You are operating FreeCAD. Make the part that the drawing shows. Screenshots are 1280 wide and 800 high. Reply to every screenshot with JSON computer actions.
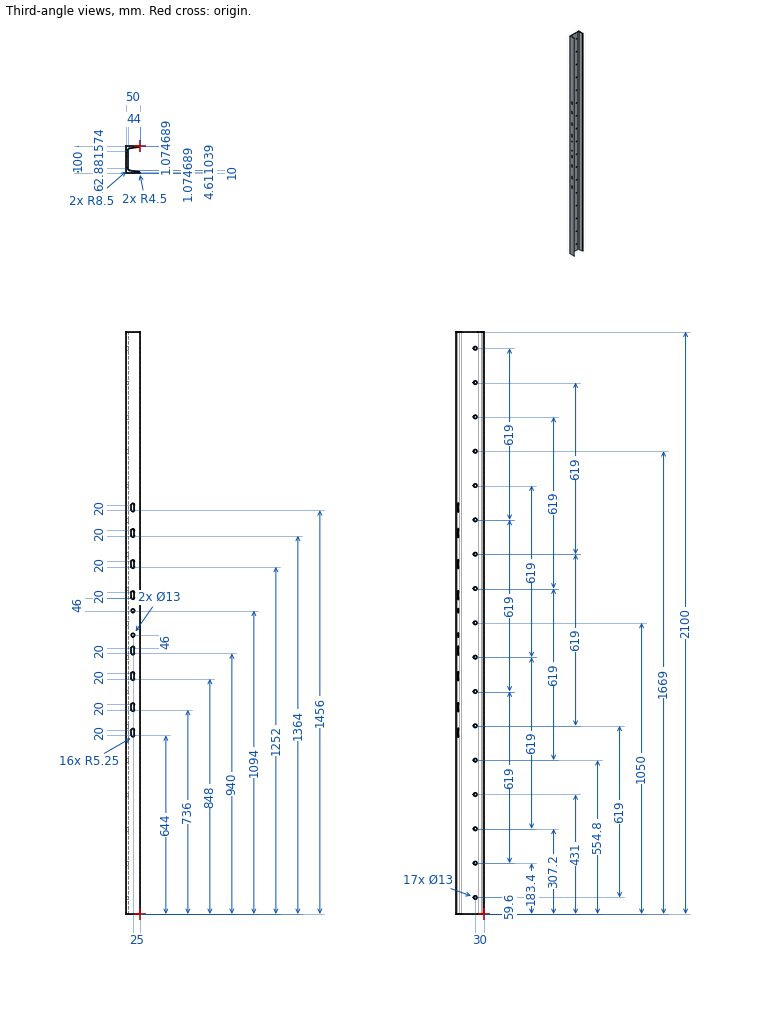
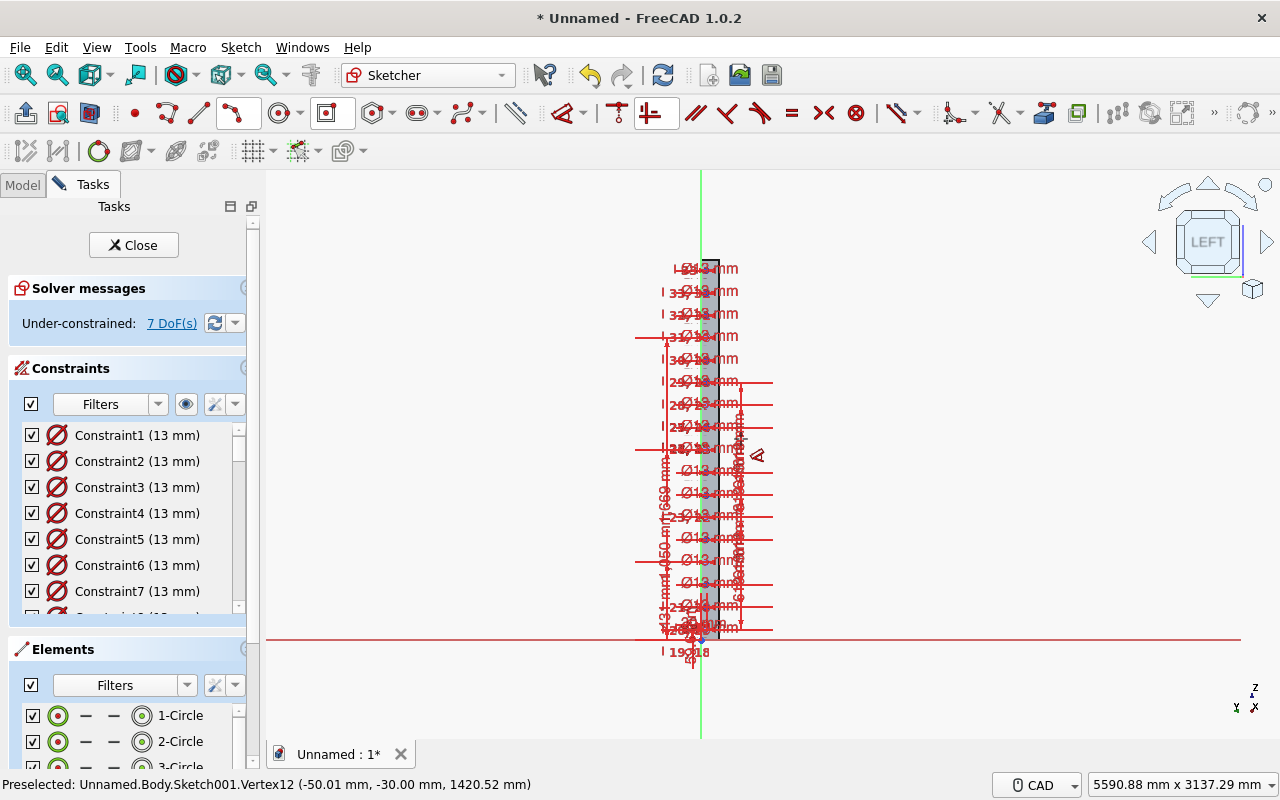
{"action": "left_click", "coordinate": [707, 473]}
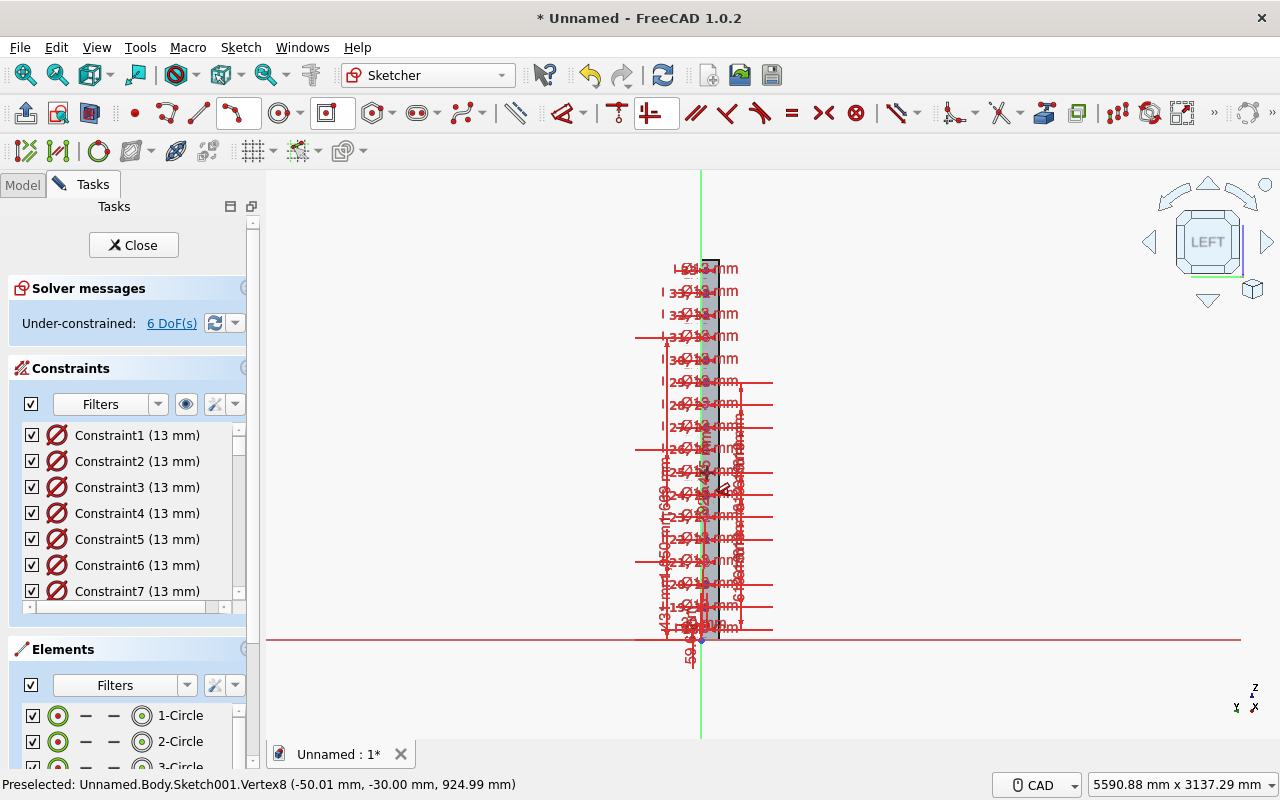
{"action": "left_click", "coordinate": [707, 361]}
{"action": "left_click", "coordinate": [741, 417]}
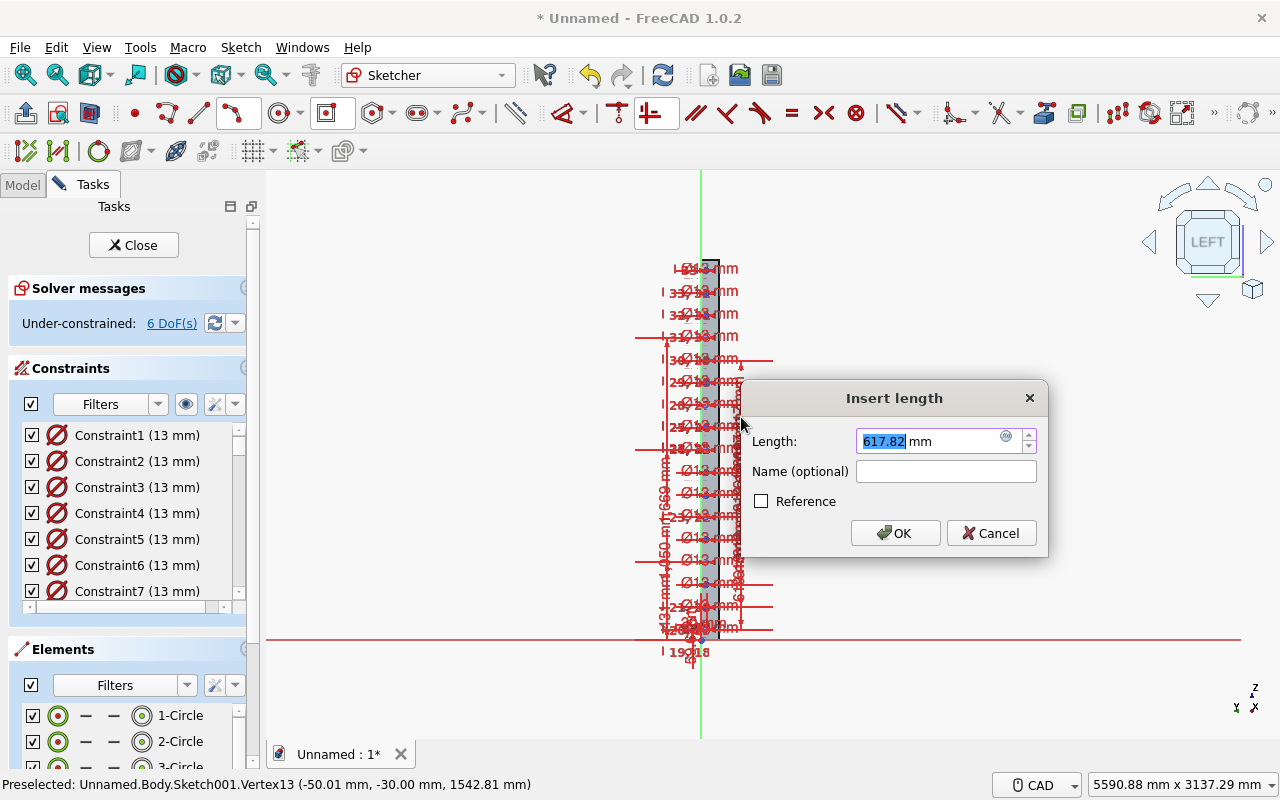
{"action": "type", "text": "619"}
{"action": "key", "text": "Return"}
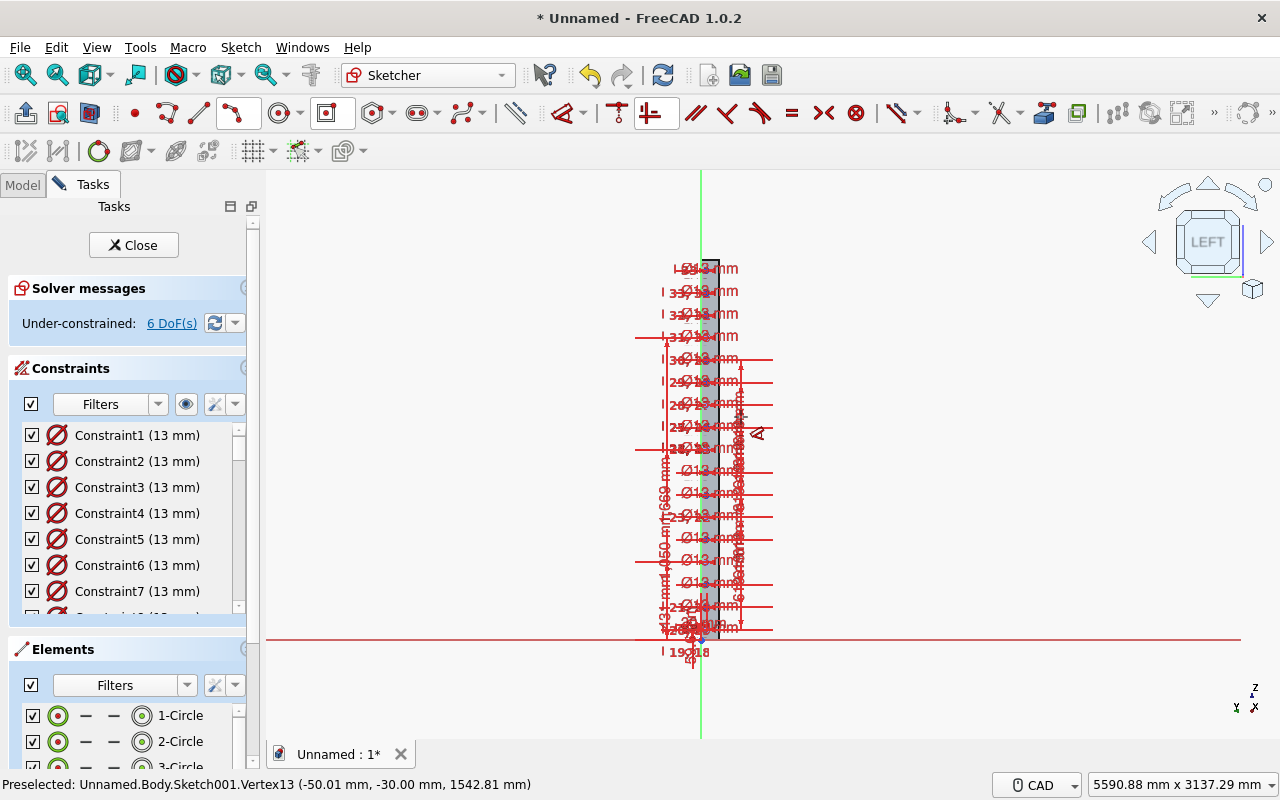
{"action": "left_click", "coordinate": [707, 428]}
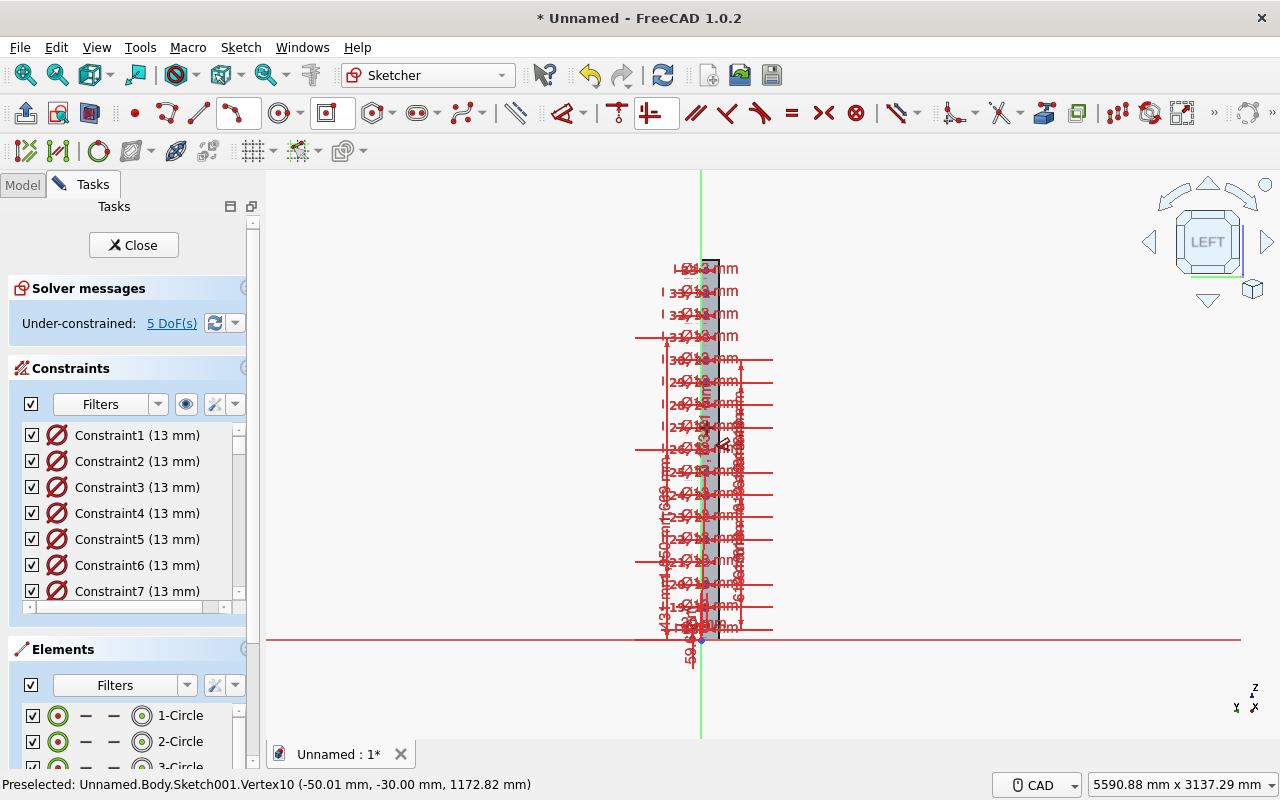
{"action": "left_click", "coordinate": [707, 316]}
{"action": "left_click", "coordinate": [741, 372]}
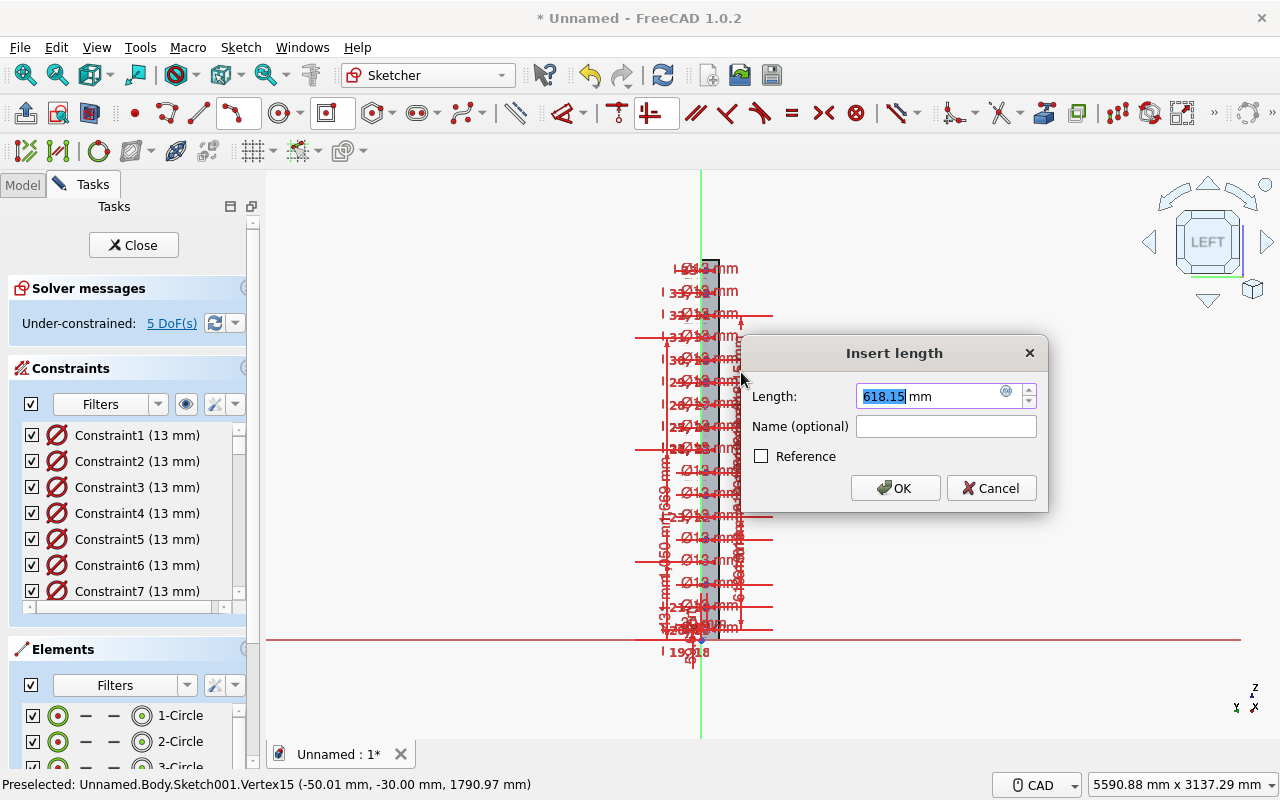
{"action": "type", "text": "619"}
{"action": "key", "text": "Return"}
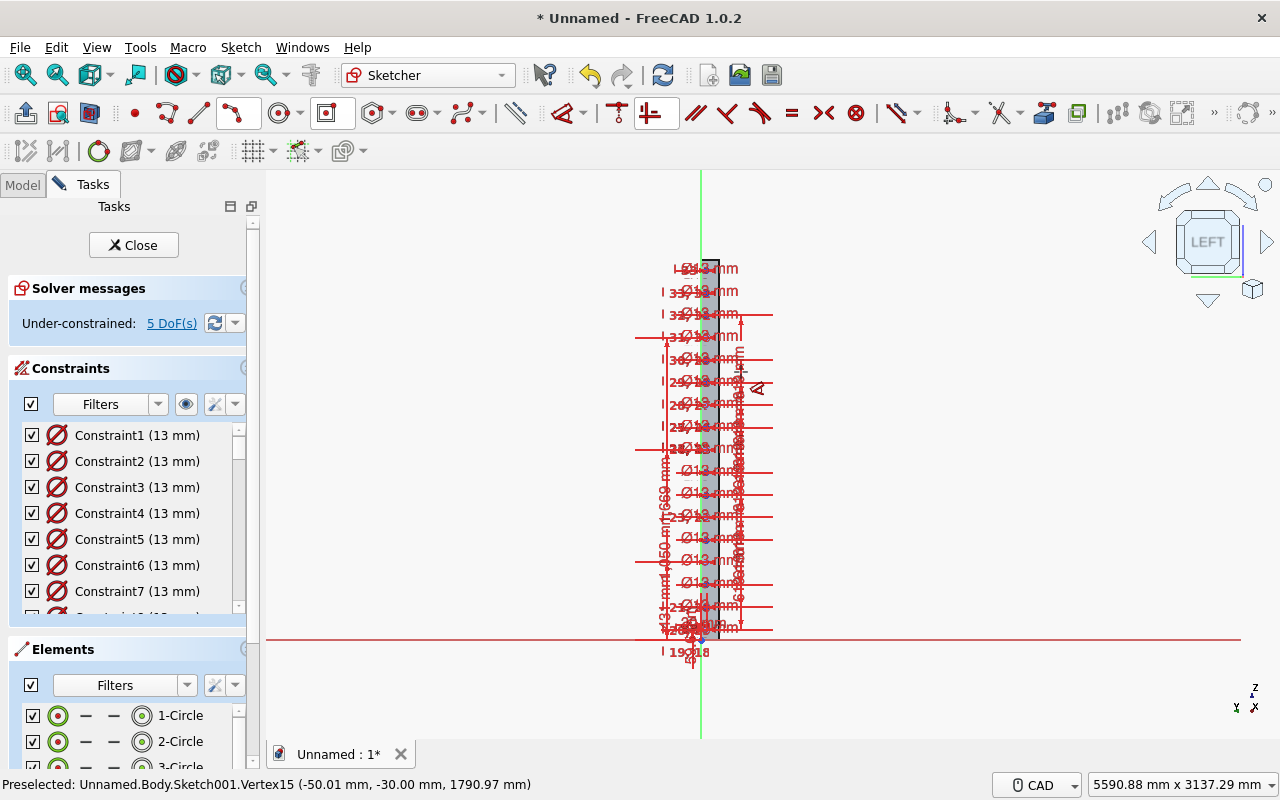
{"action": "left_click", "coordinate": [707, 405]}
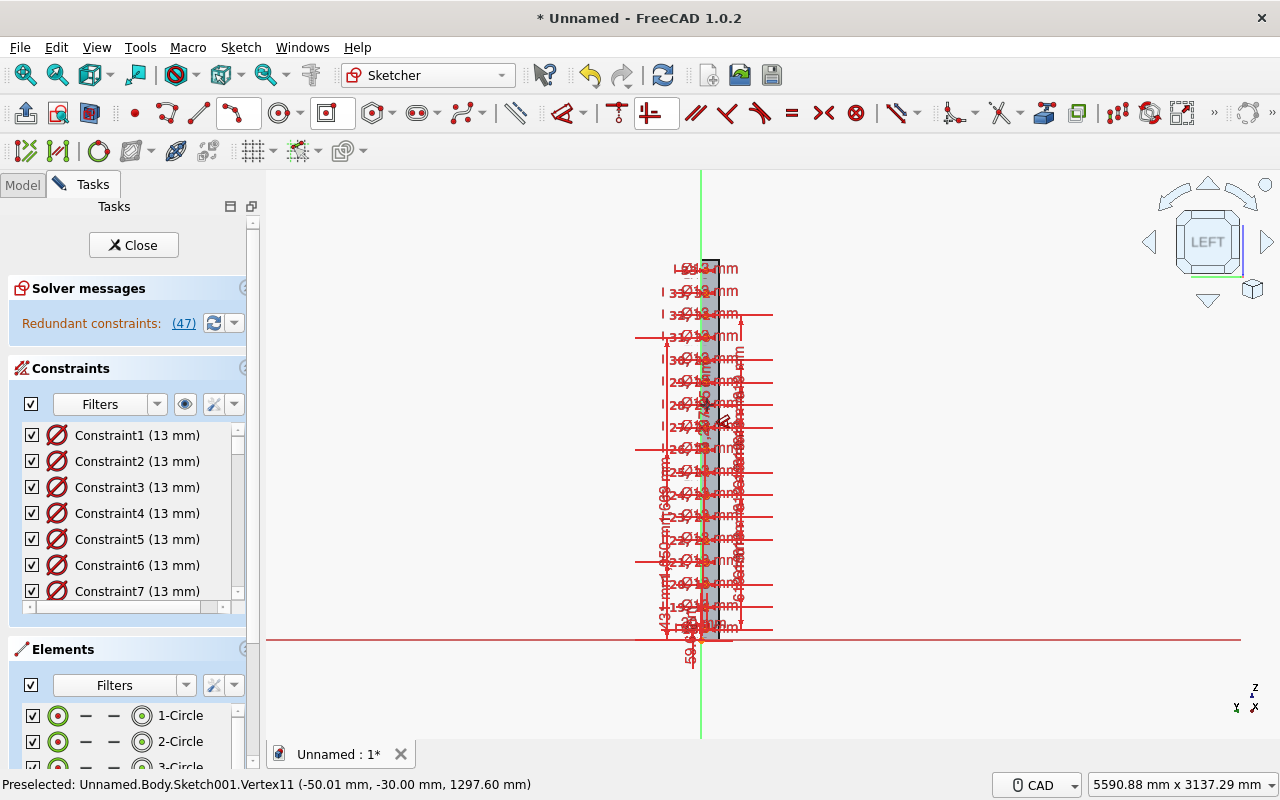
{"action": "left_click", "coordinate": [707, 293]}
{"action": "left_click", "coordinate": [741, 349]}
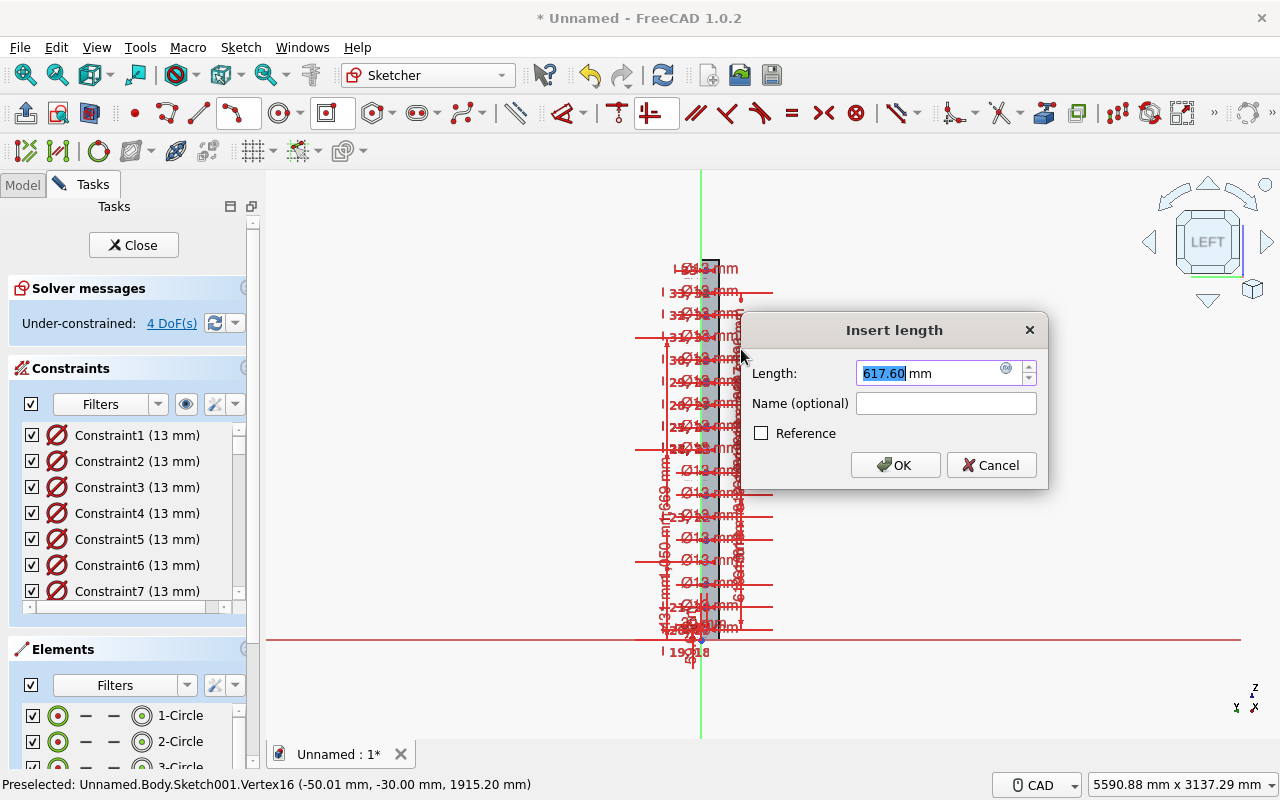
{"action": "type", "text": "619"}
{"action": "key", "text": "Return"}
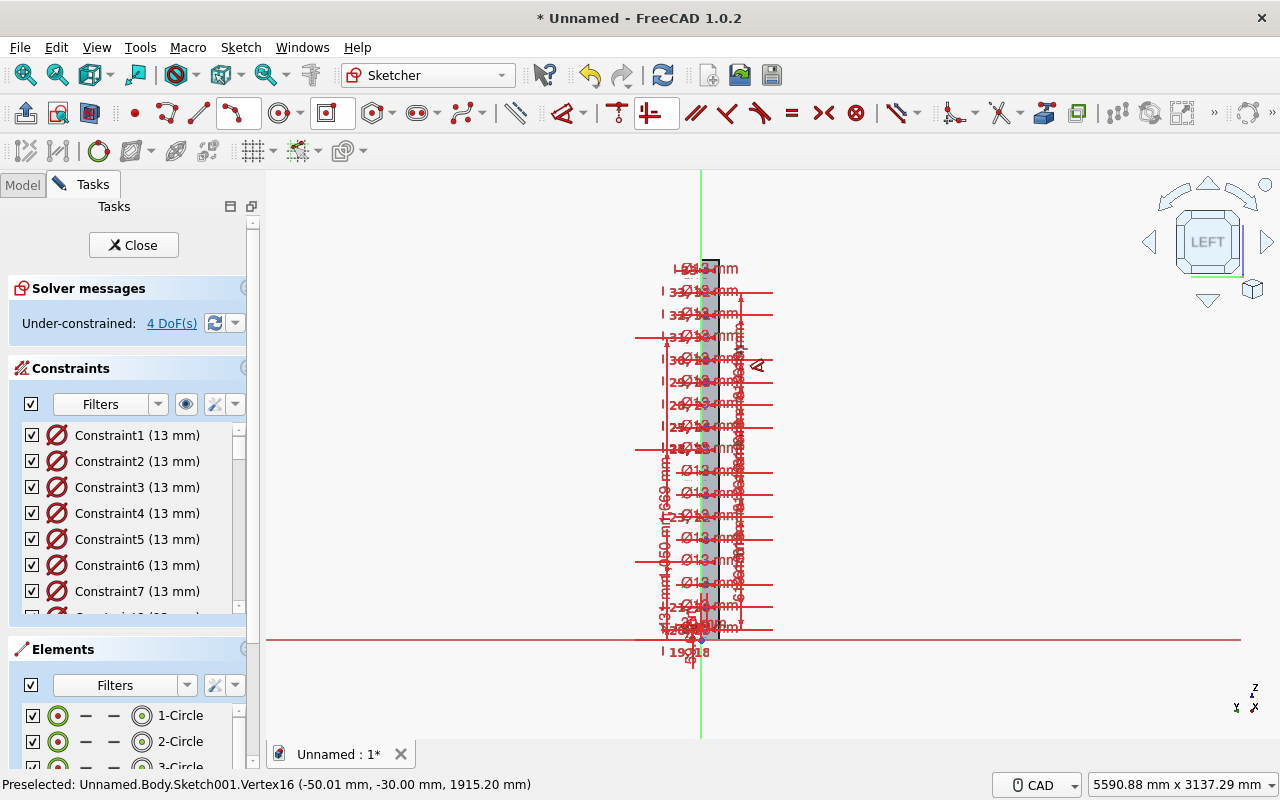
{"action": "left_click", "coordinate": [707, 383]}